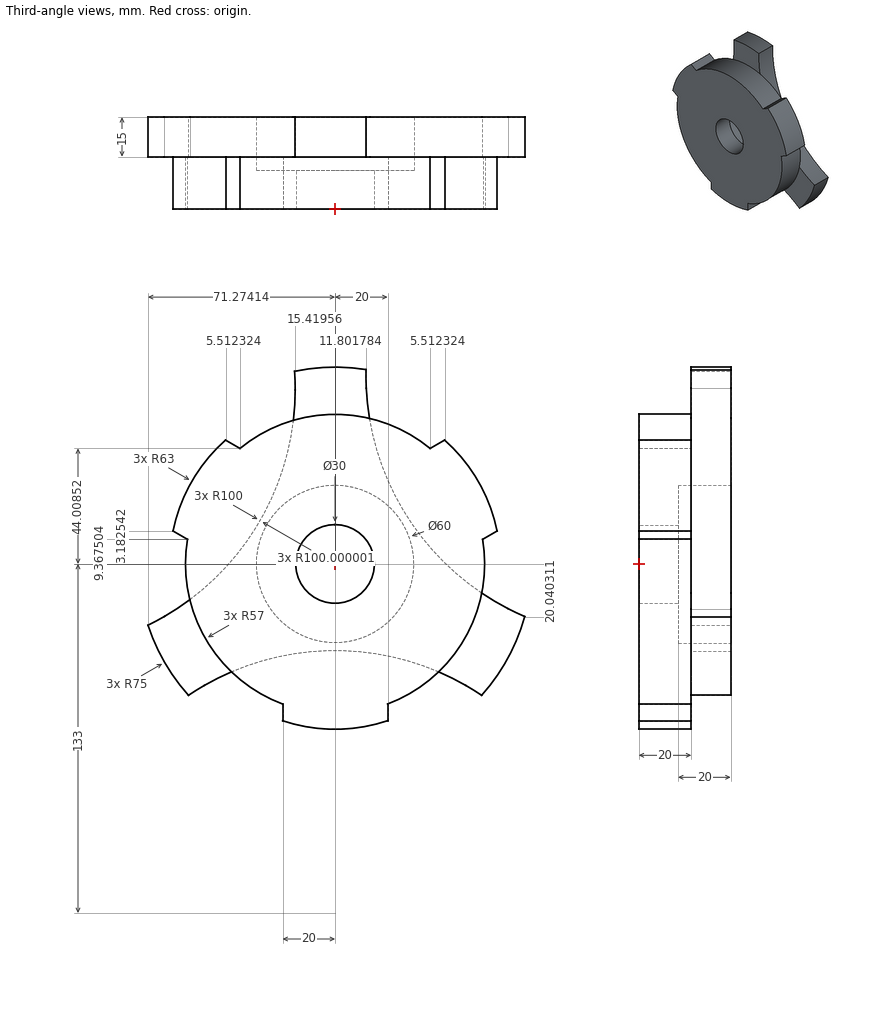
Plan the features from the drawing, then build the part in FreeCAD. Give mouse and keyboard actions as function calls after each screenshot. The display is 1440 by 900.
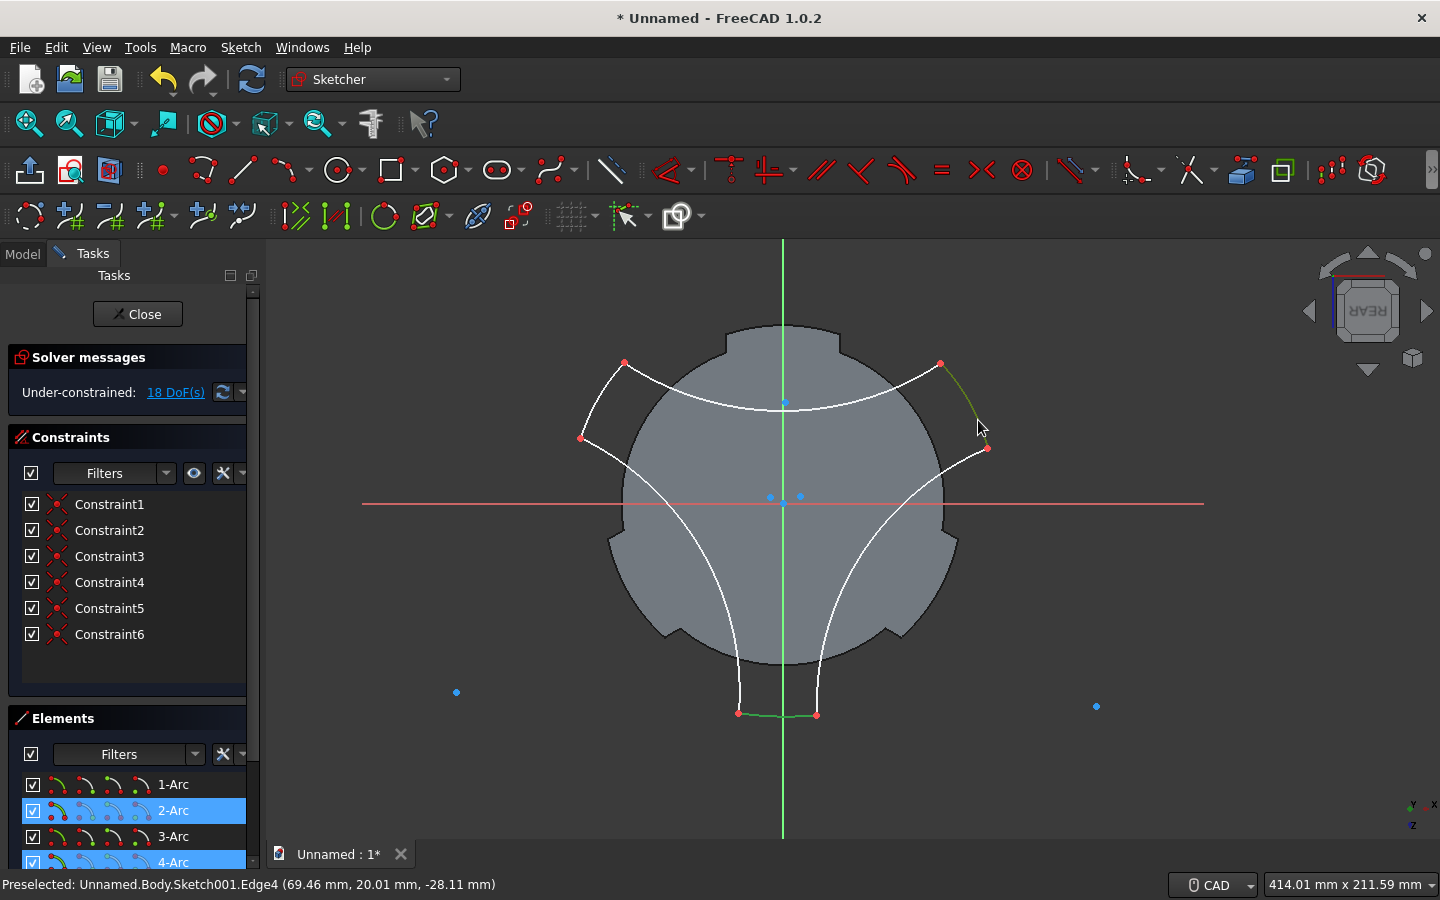
key(c)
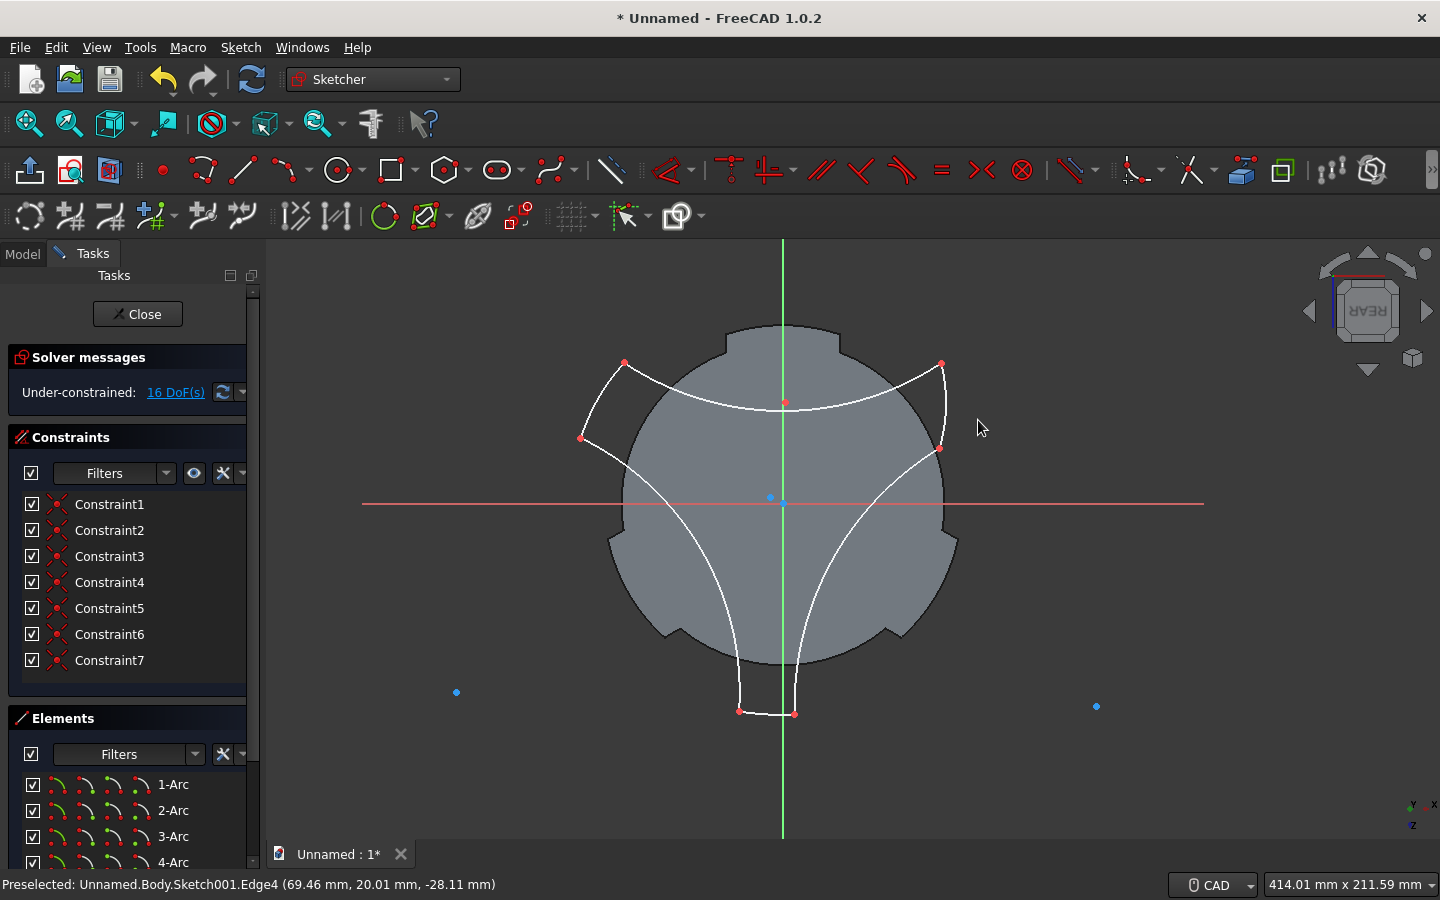
click(756, 714)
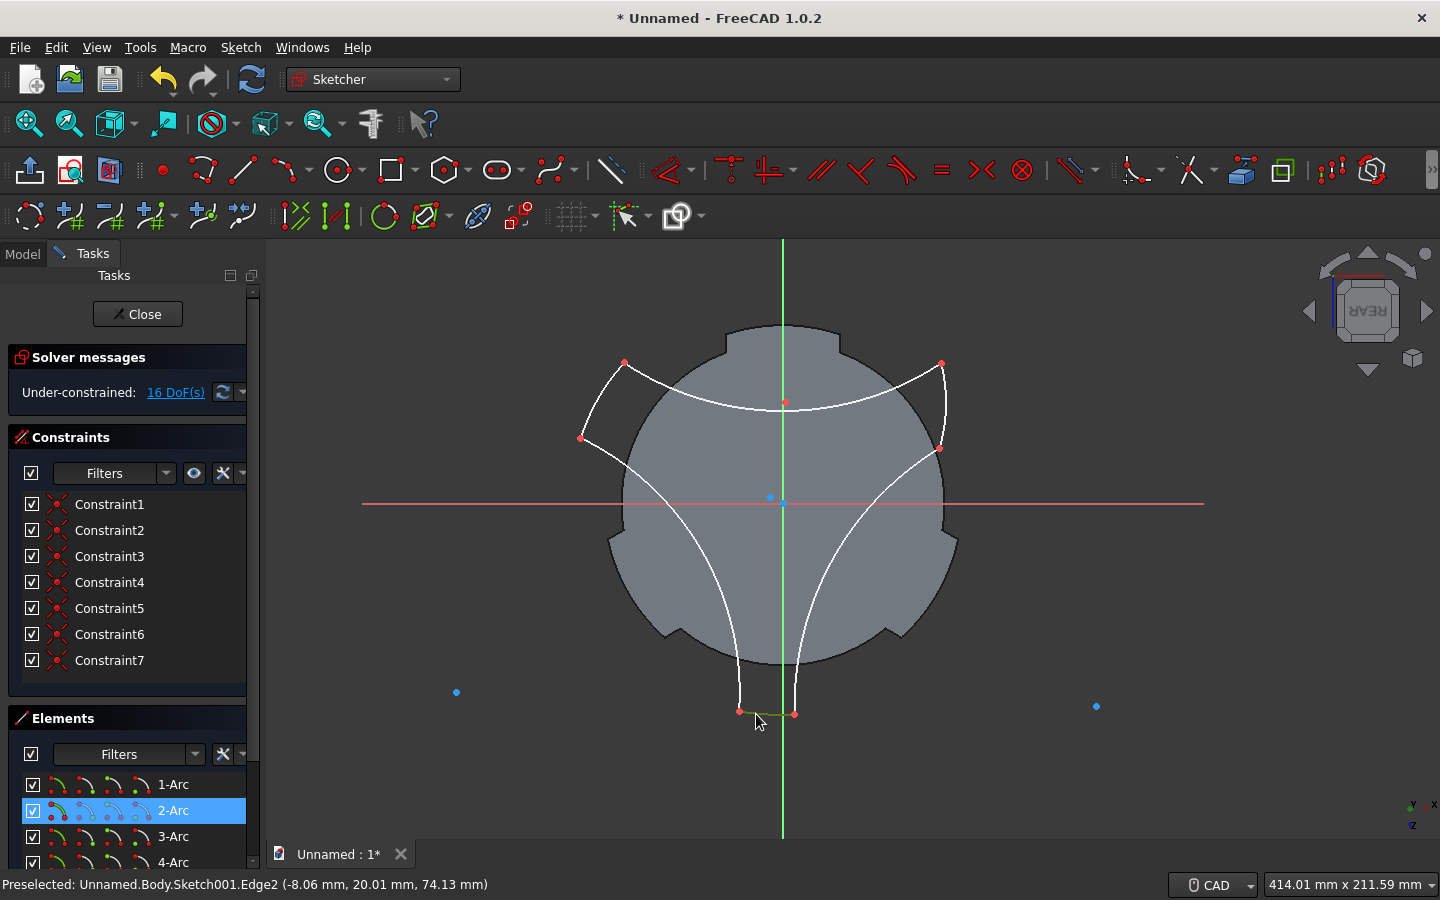
click(608, 383)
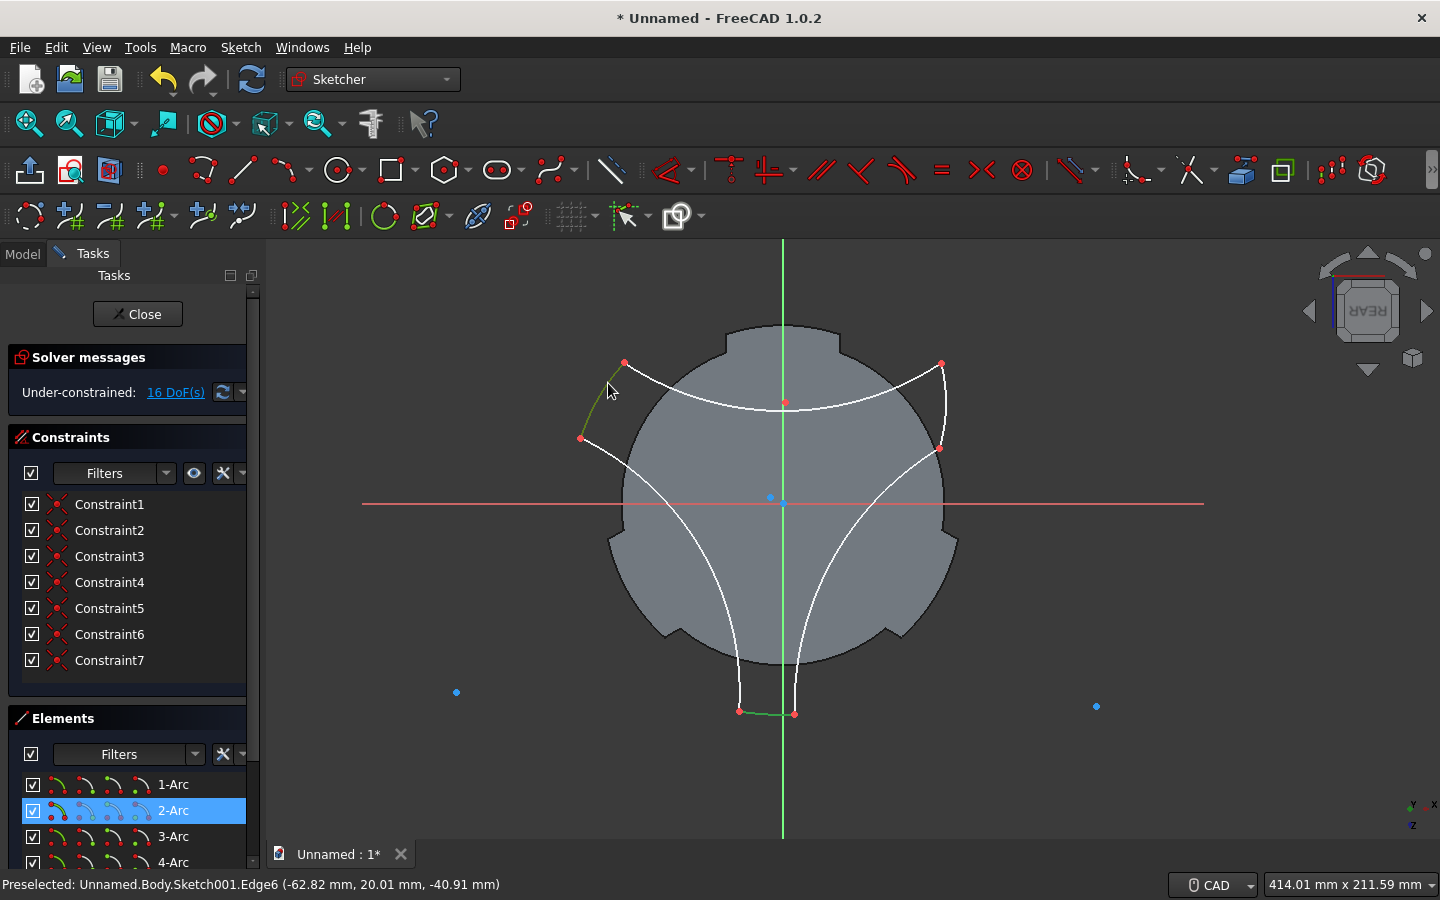
click(730, 170)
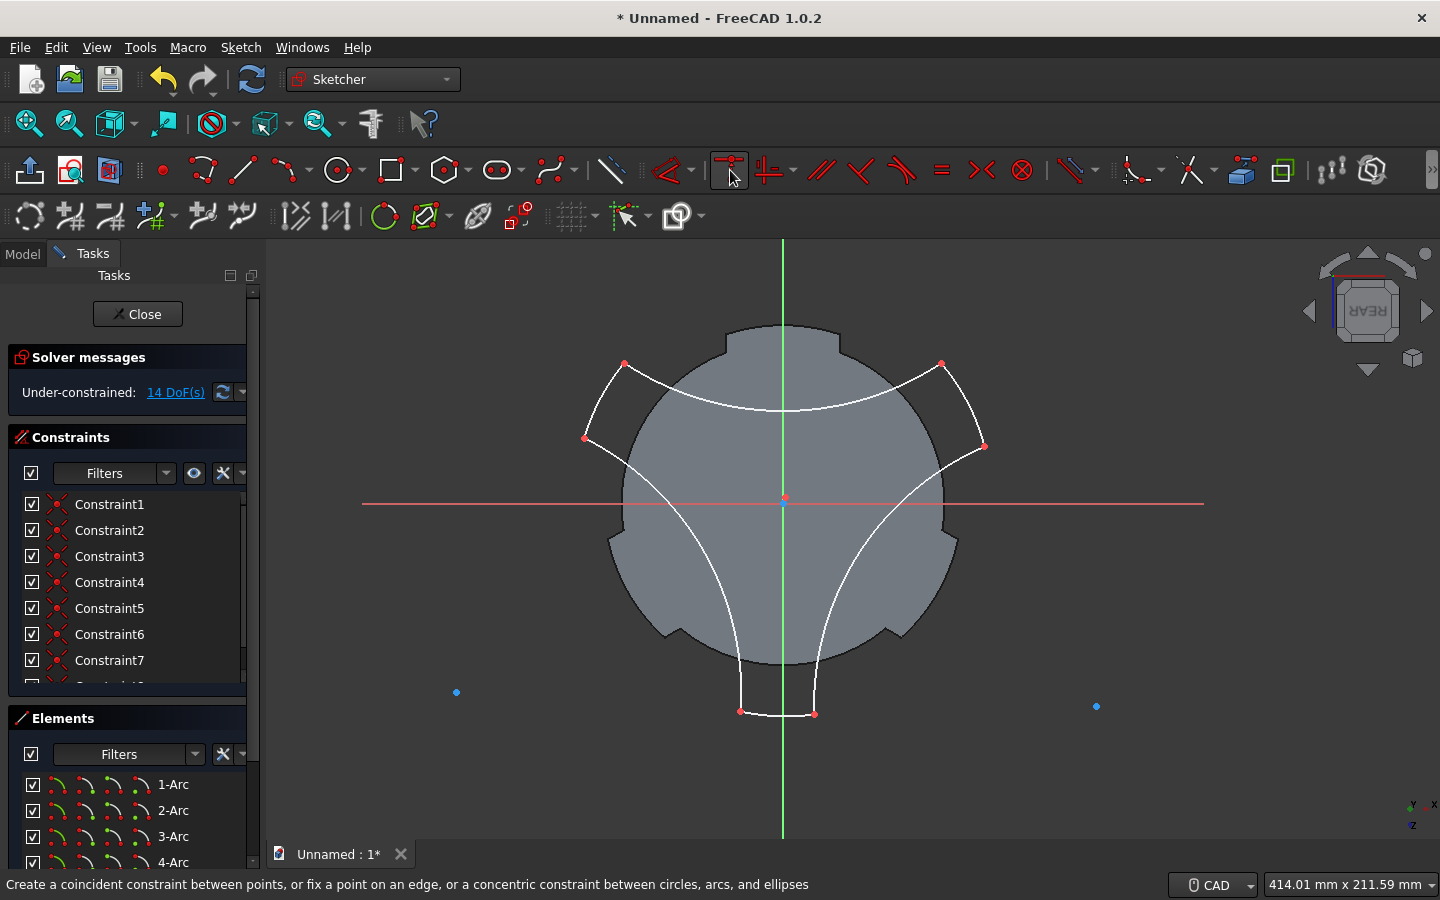
drag(773, 487, 796, 514)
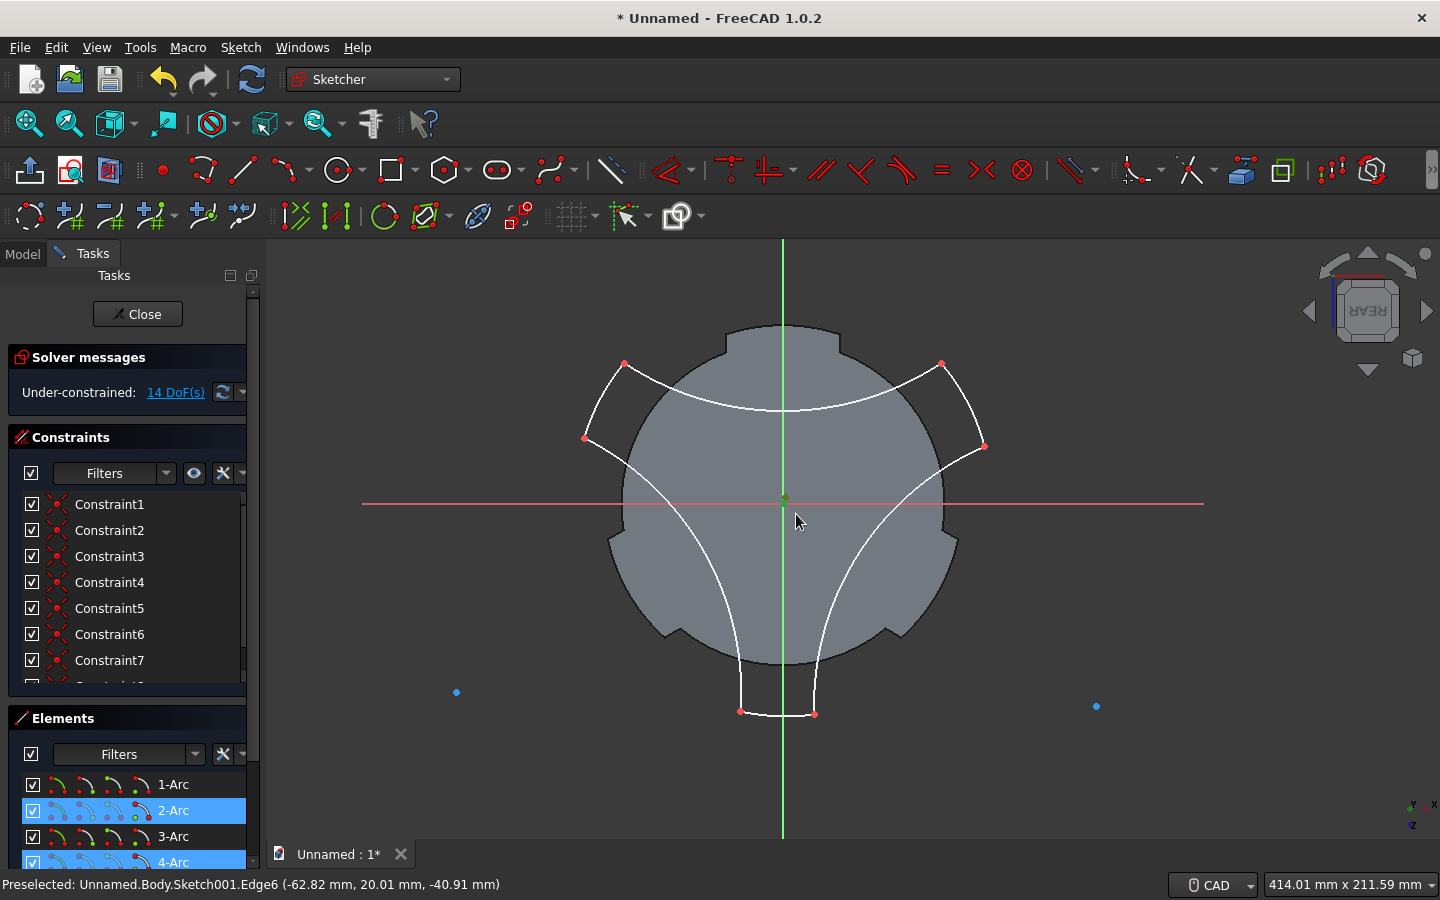
click(730, 170)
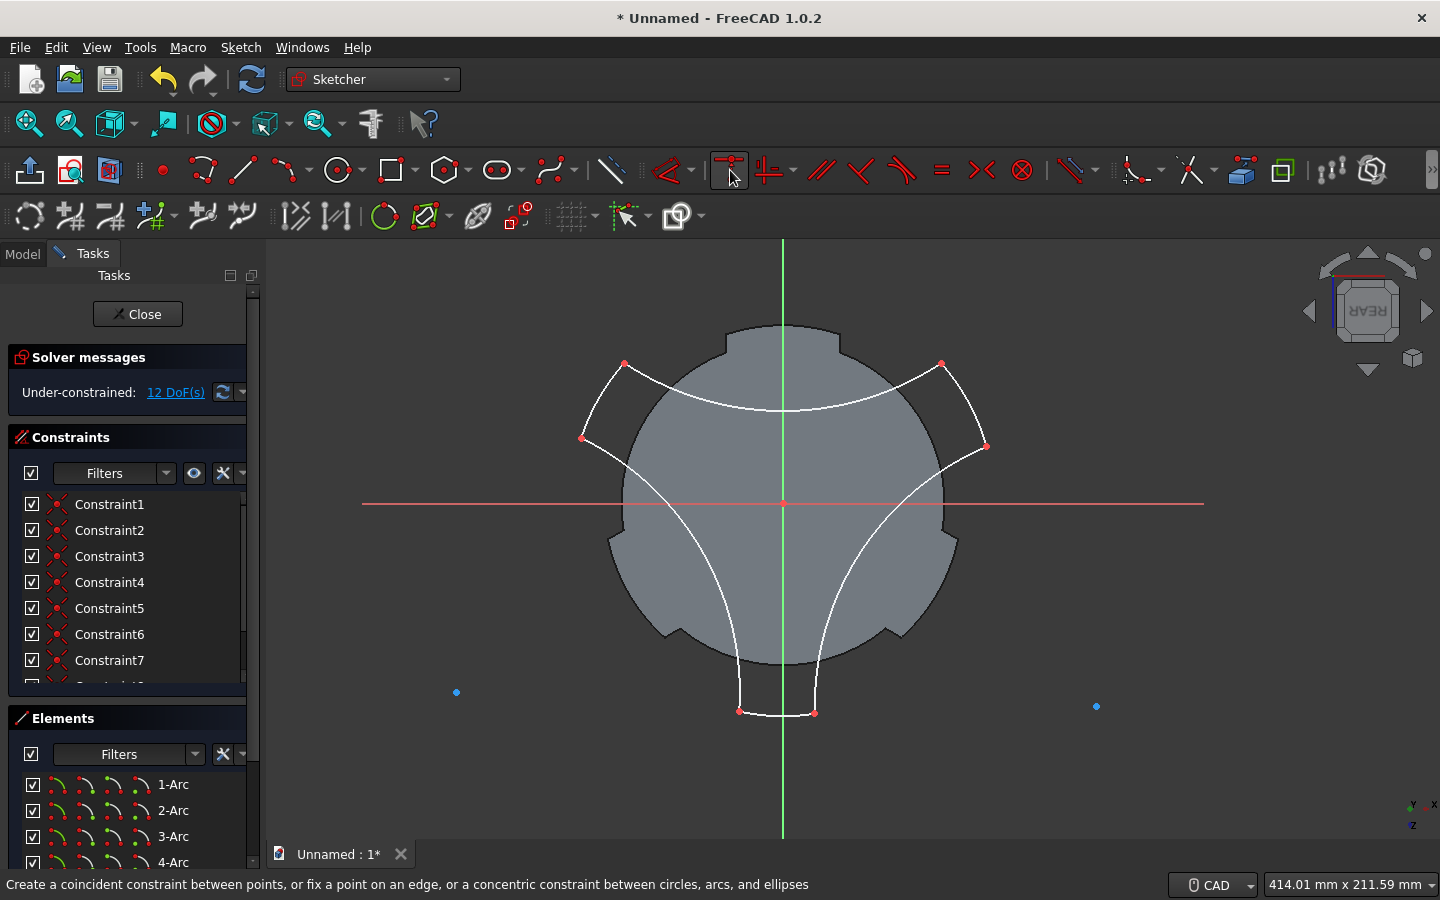
click(762, 715)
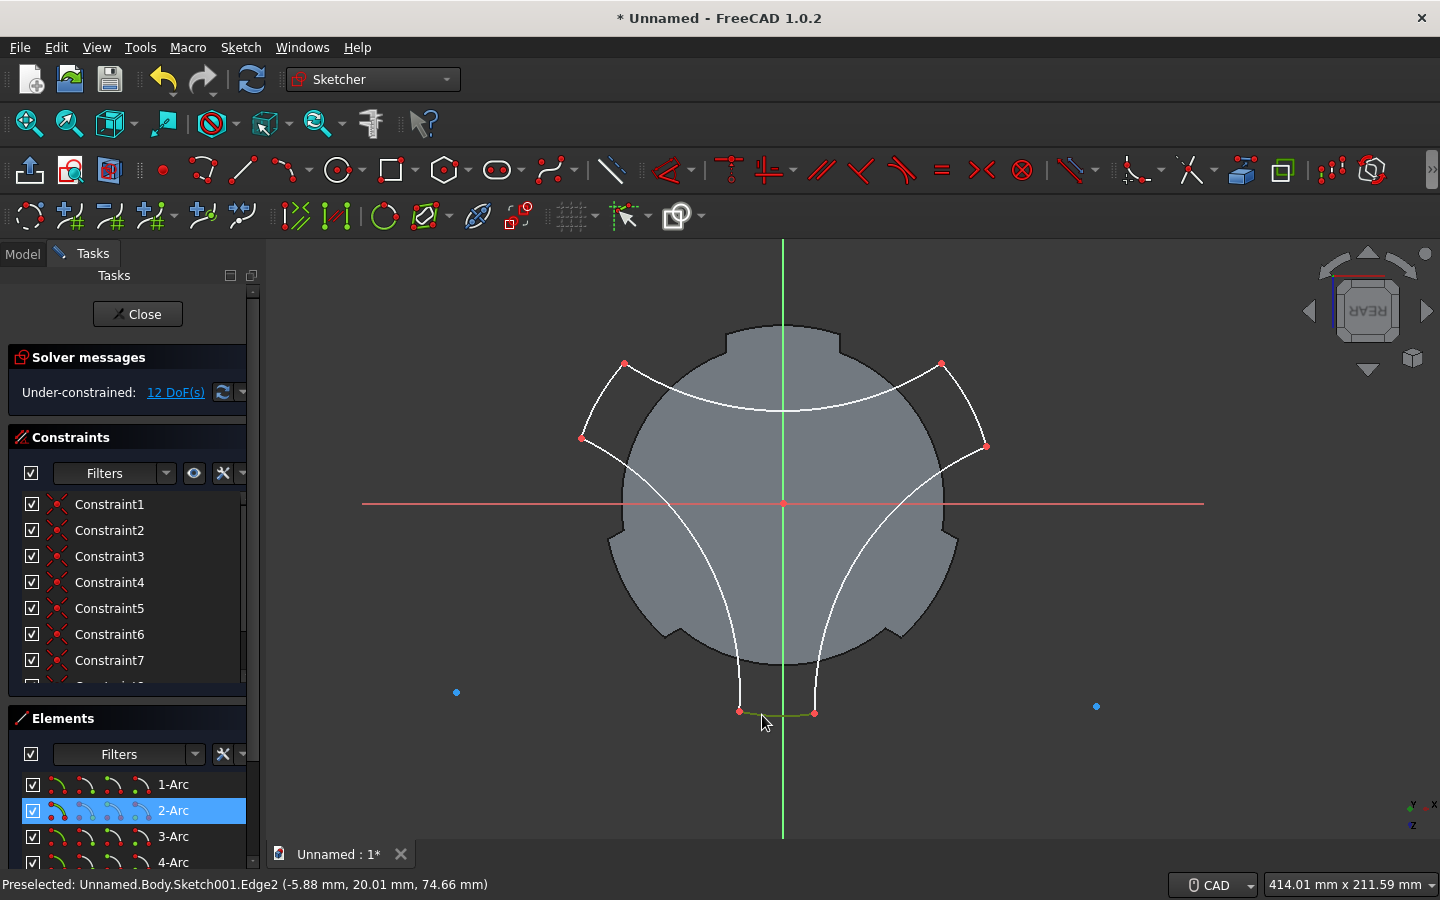
click(977, 420)